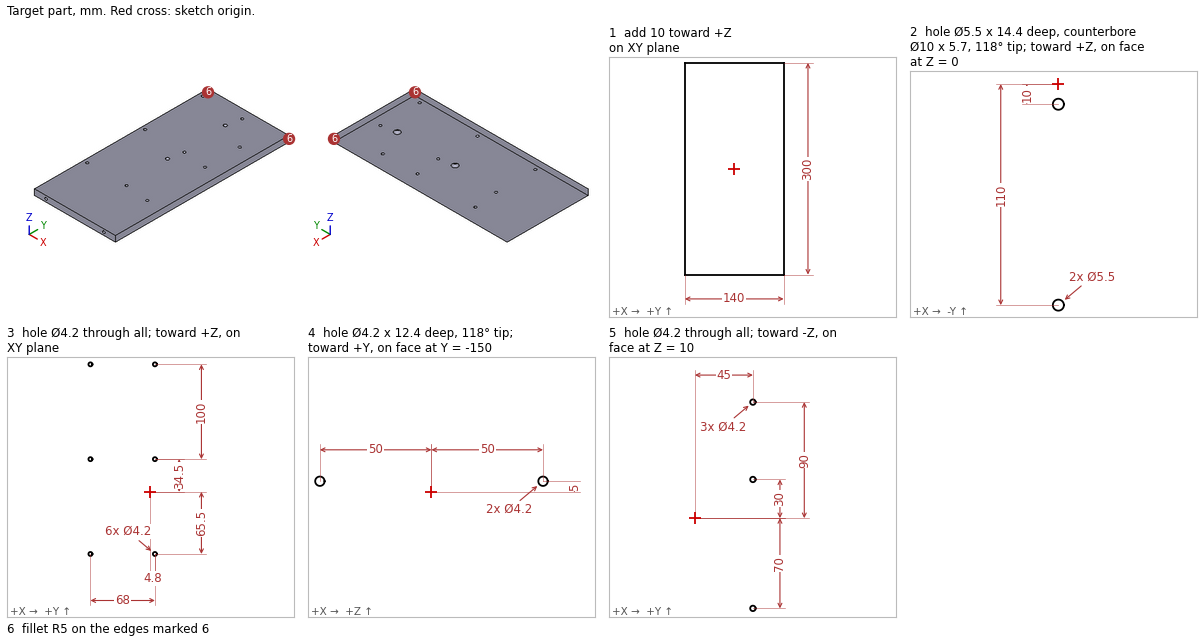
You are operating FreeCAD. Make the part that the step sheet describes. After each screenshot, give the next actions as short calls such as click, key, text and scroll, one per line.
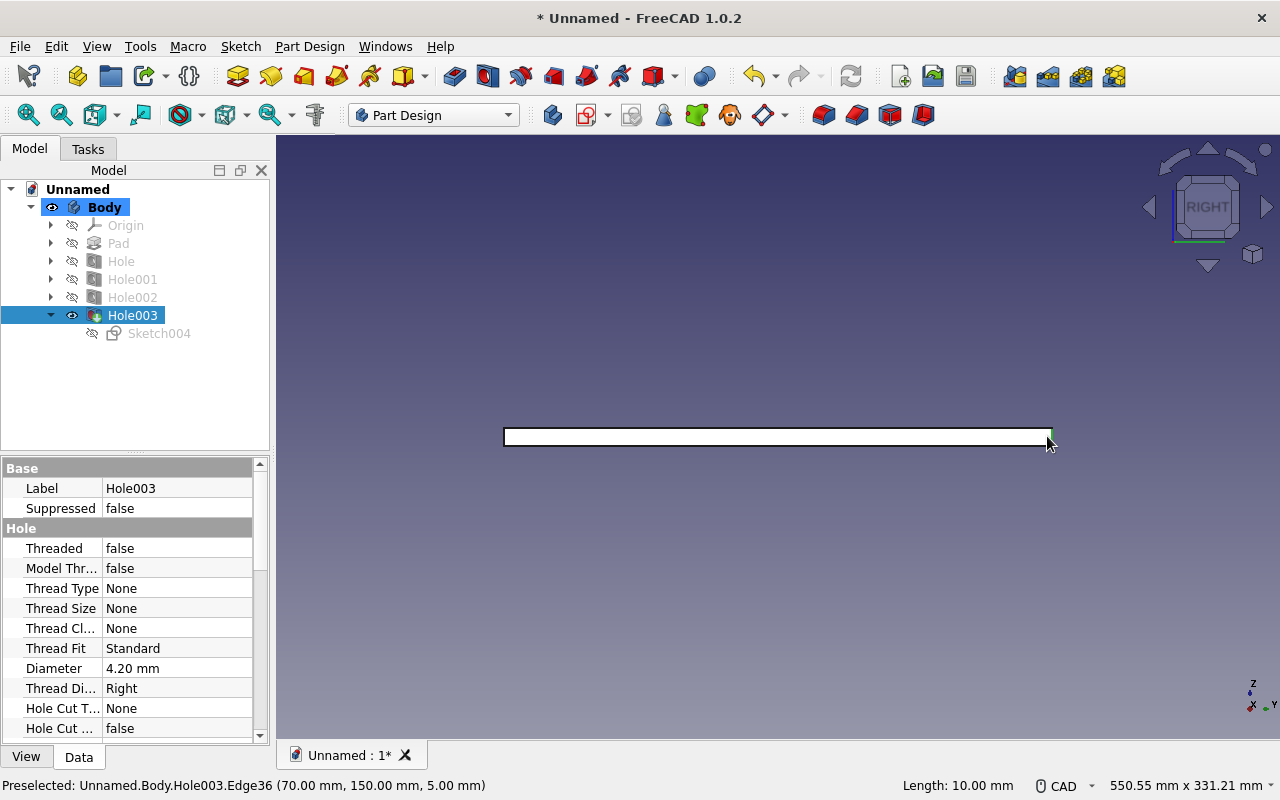
scroll(1052, 436, up, 4)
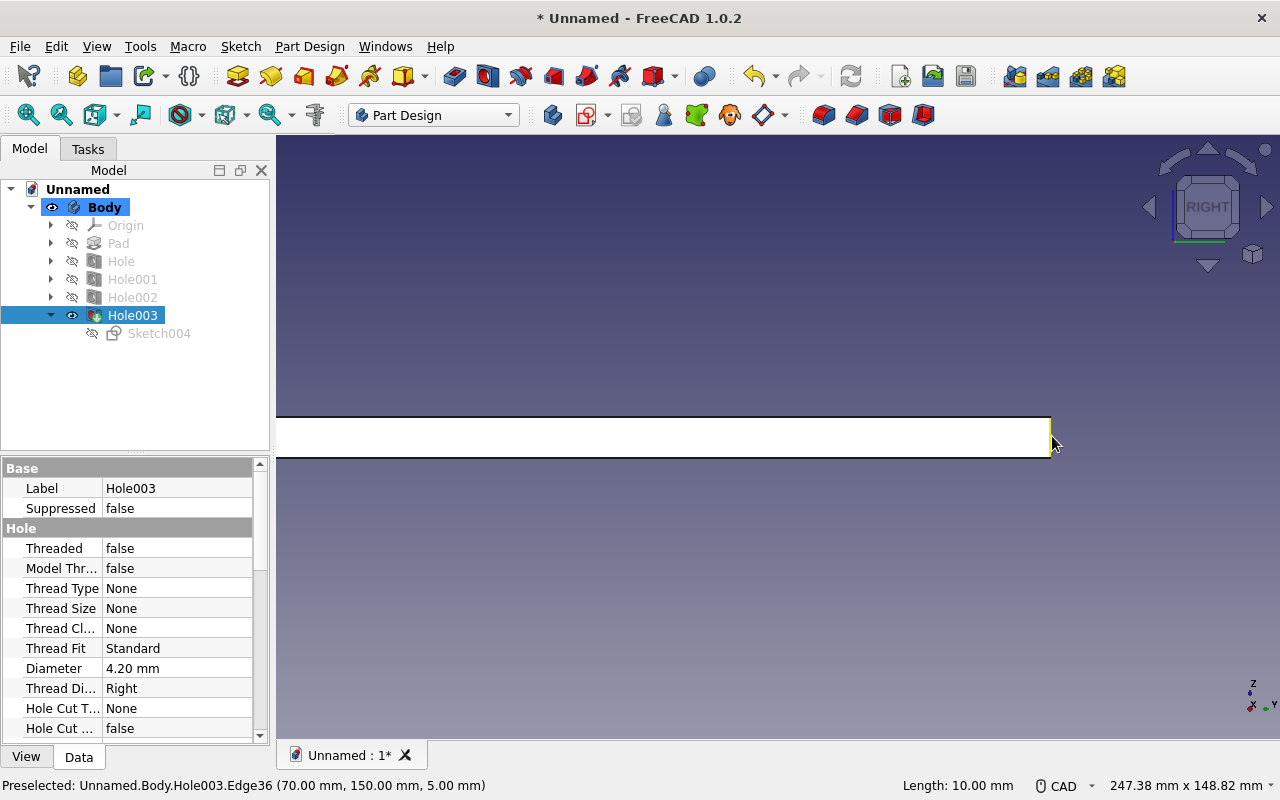
click(29, 116)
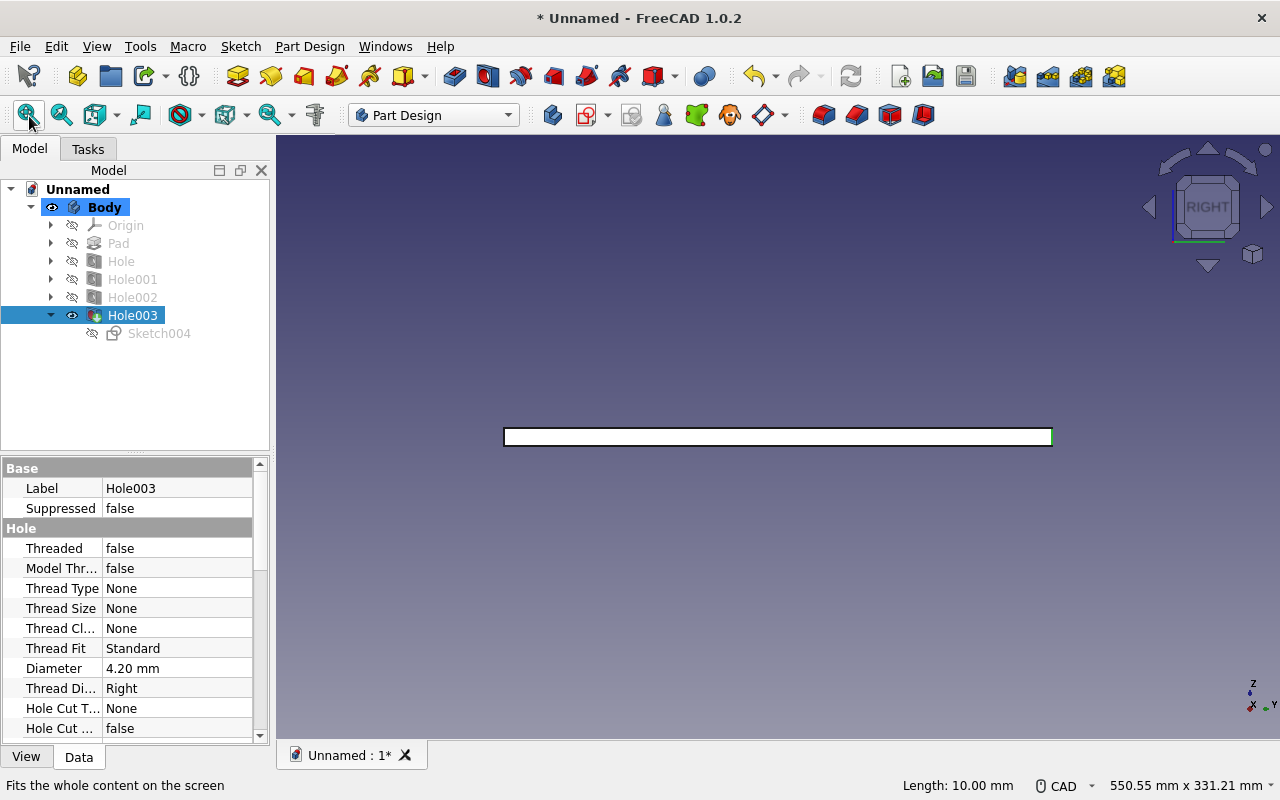
key(5)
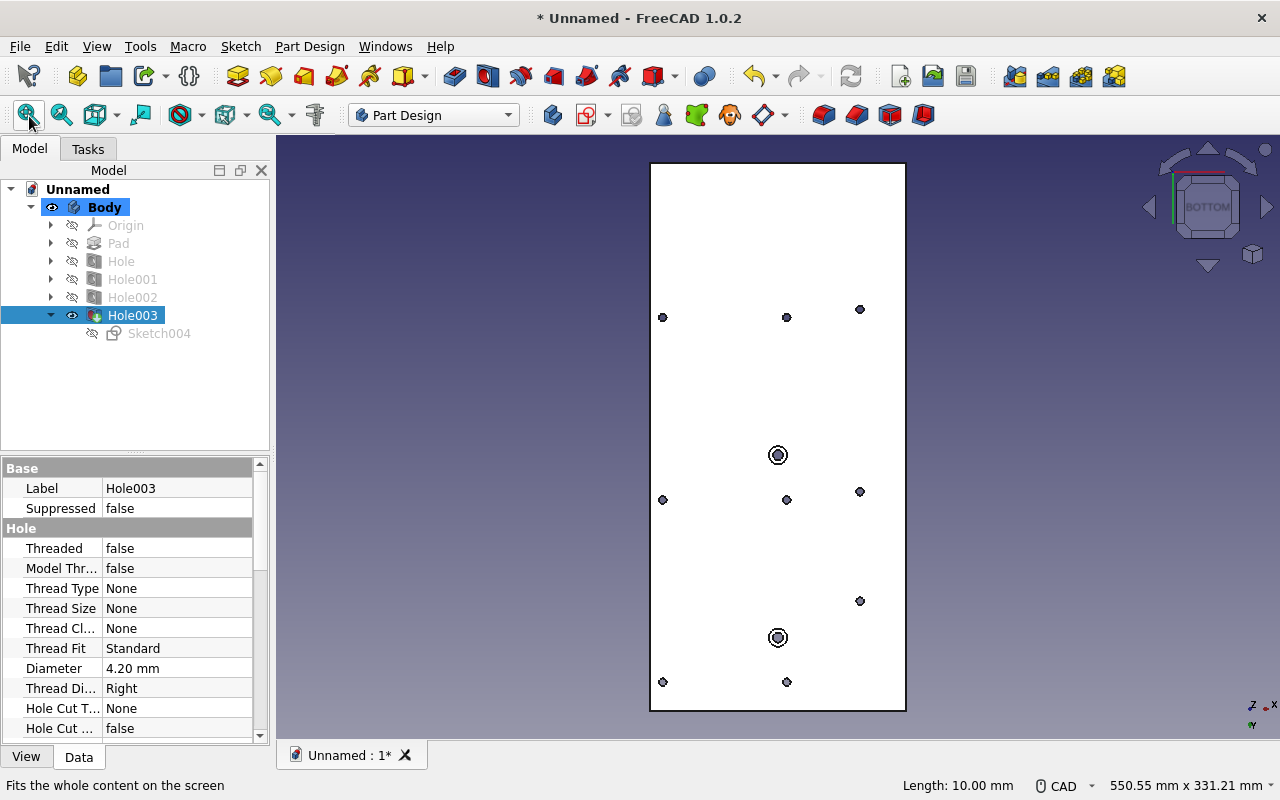
scroll(650, 710, up, 4)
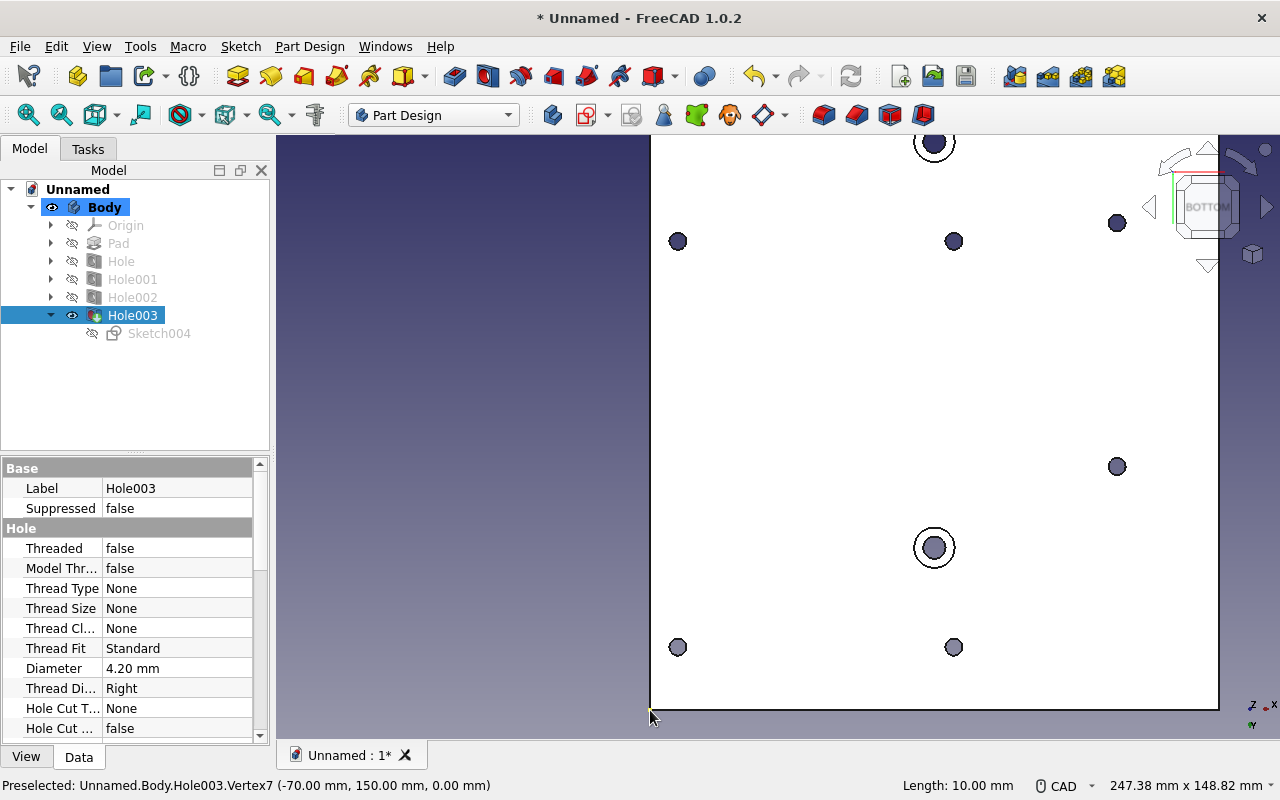
key(v)
key(f)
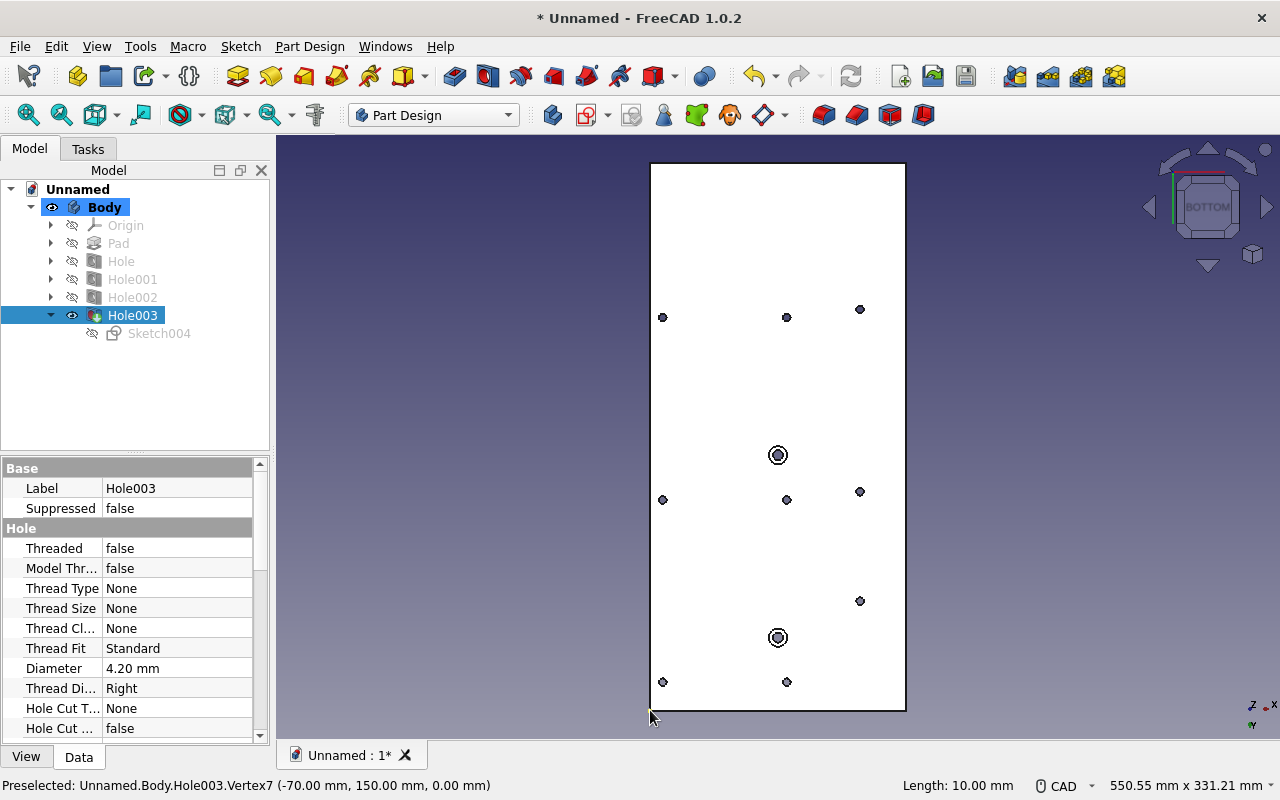
key(4)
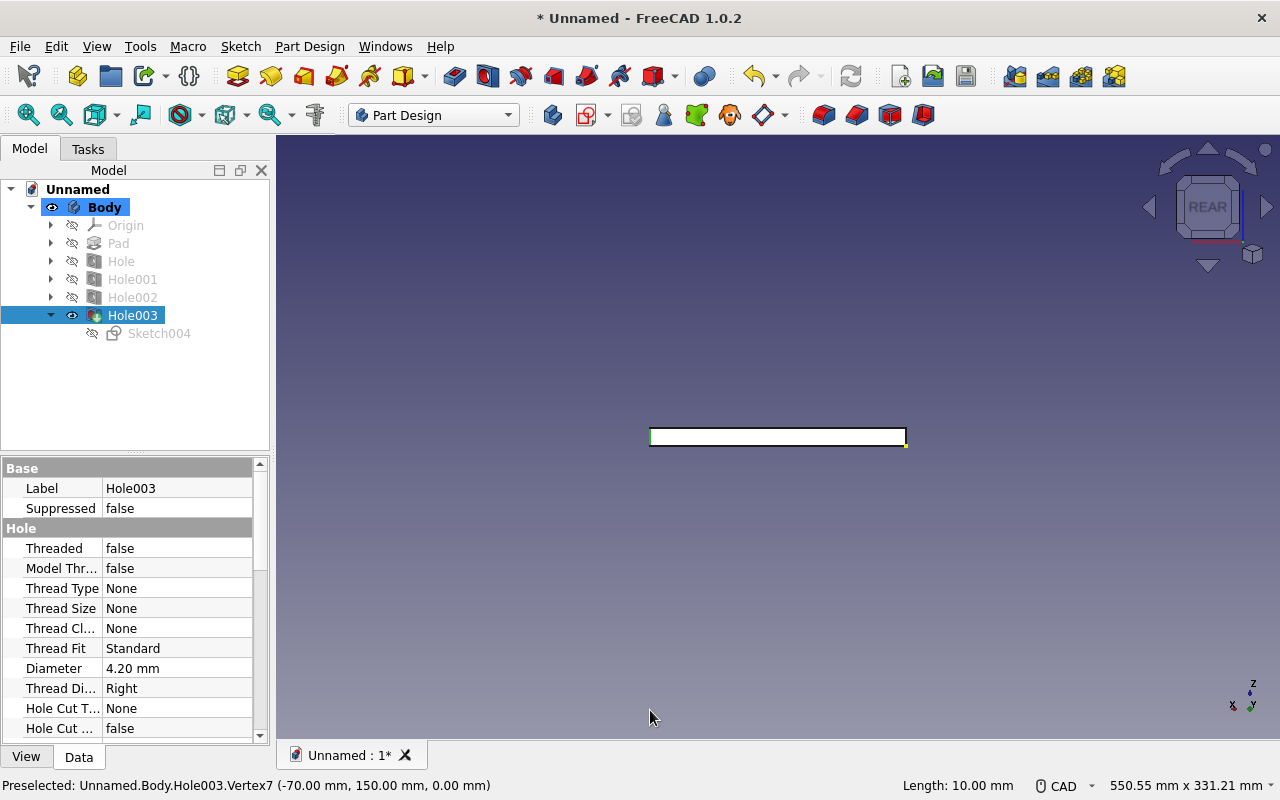
click(29, 116)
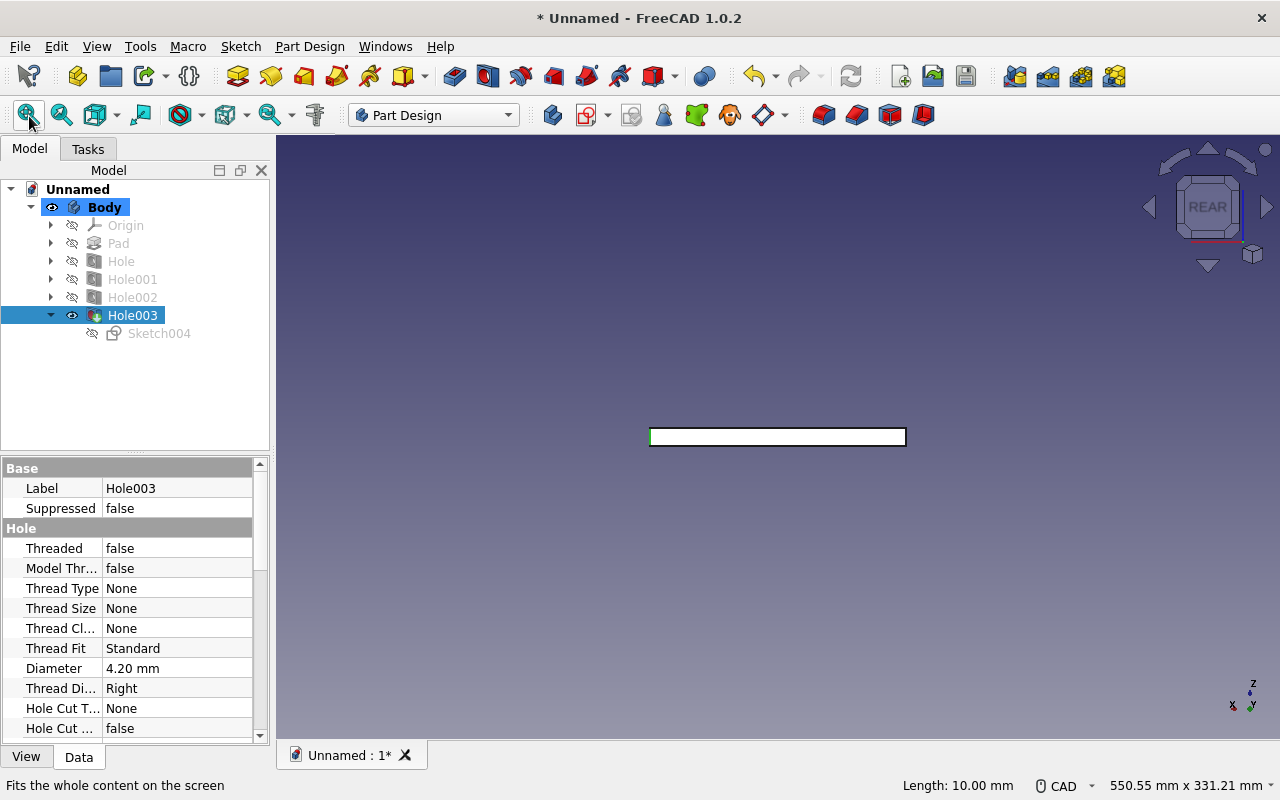
click(906, 436, ctrl)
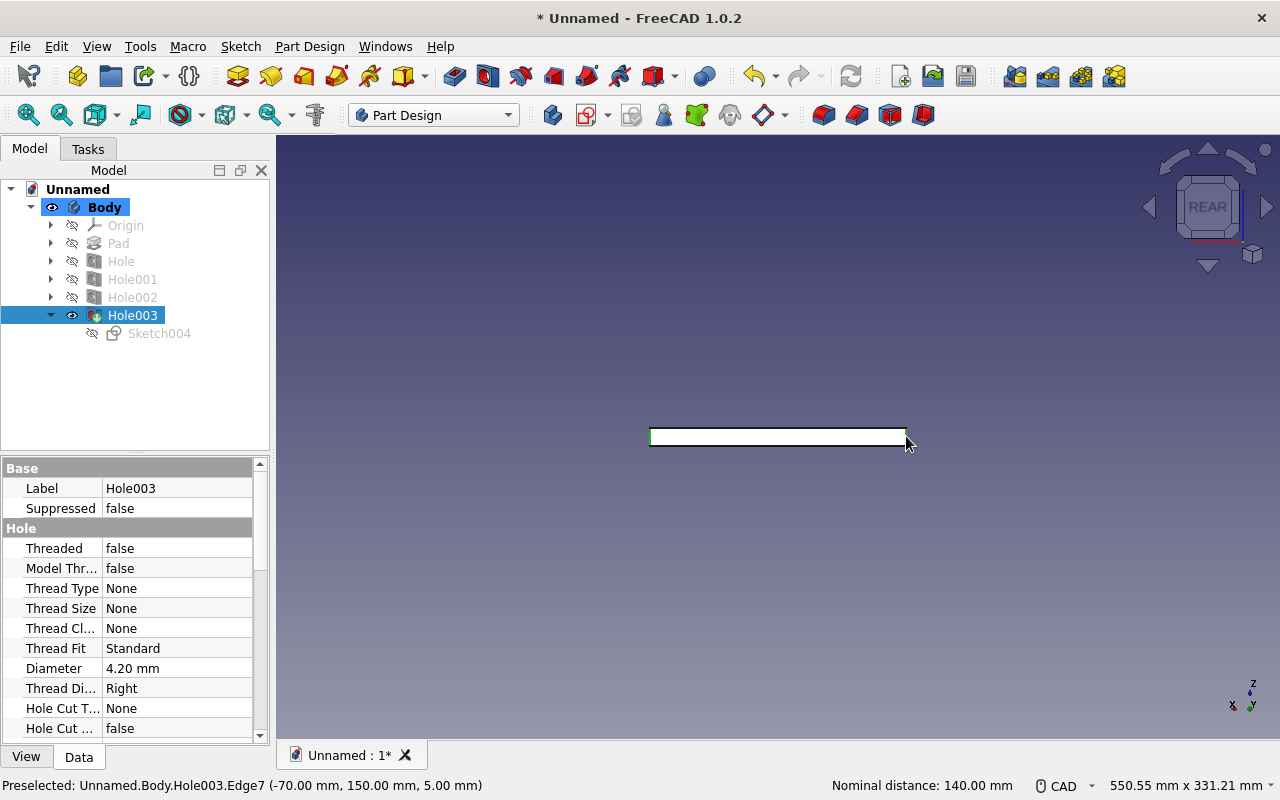
click(824, 116)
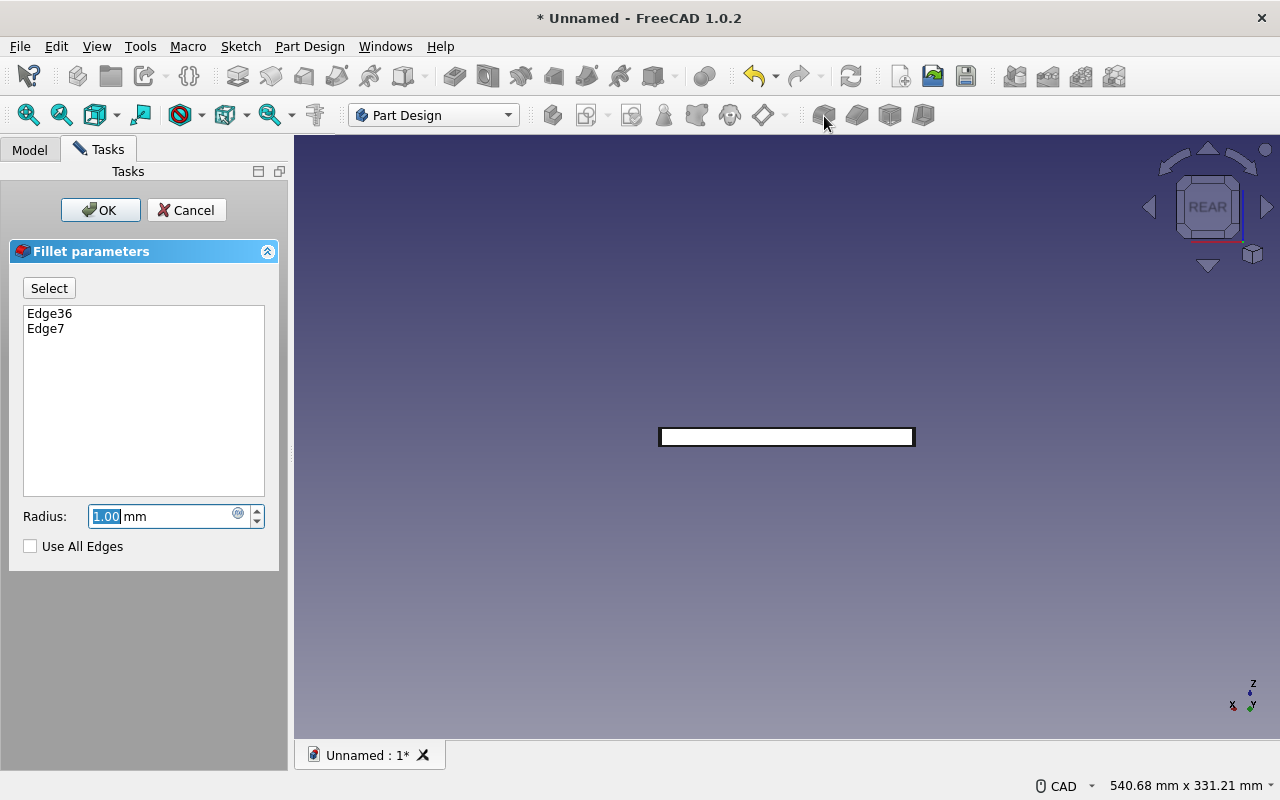
text(5)
key(Tab)